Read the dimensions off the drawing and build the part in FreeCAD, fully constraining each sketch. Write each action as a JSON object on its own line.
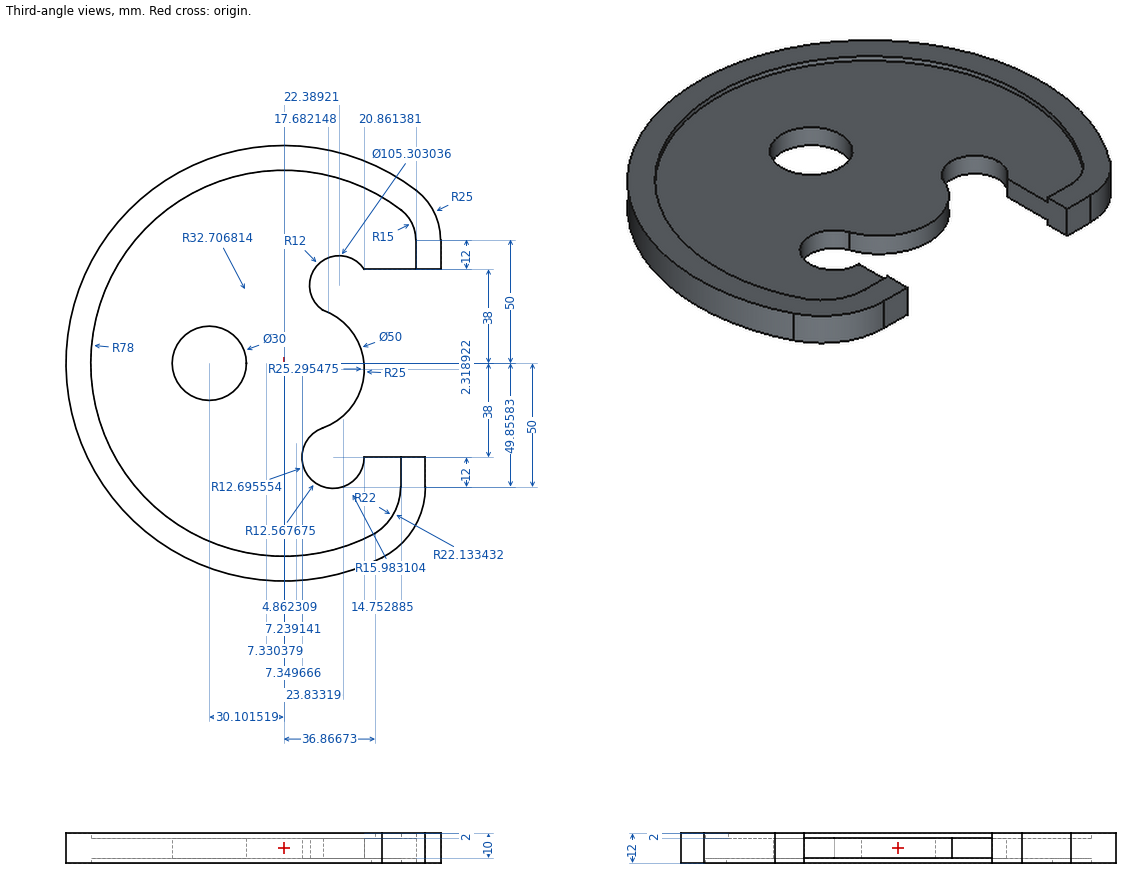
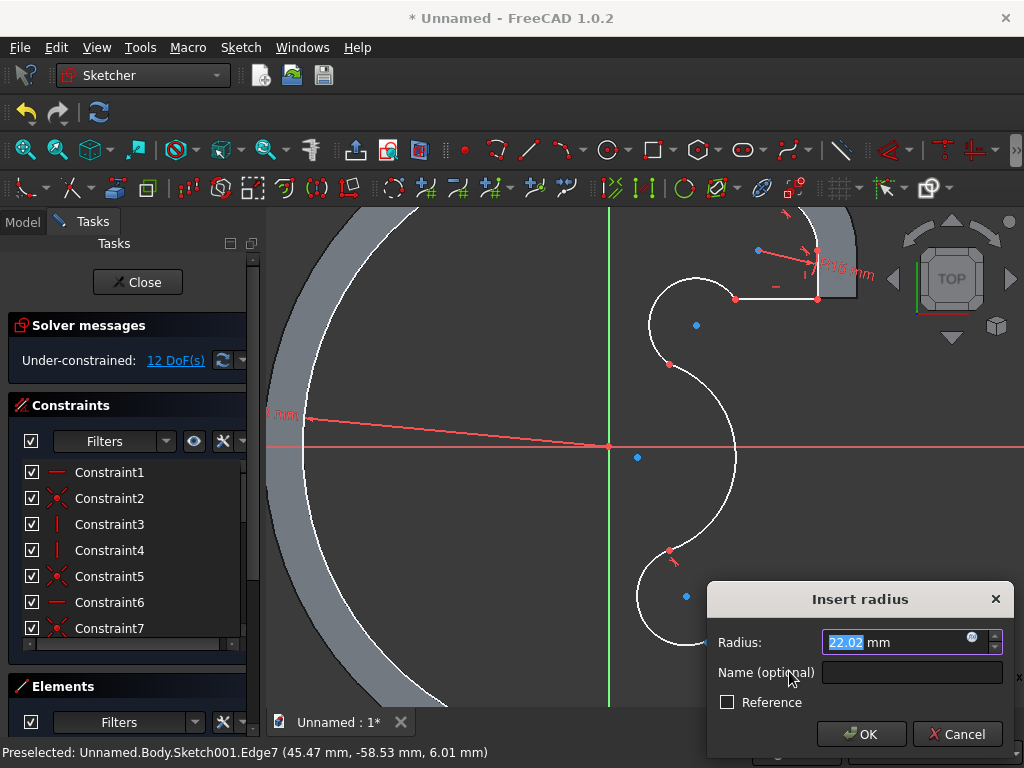
{"action": "type", "text": "22"}
{"action": "key", "text": "Return"}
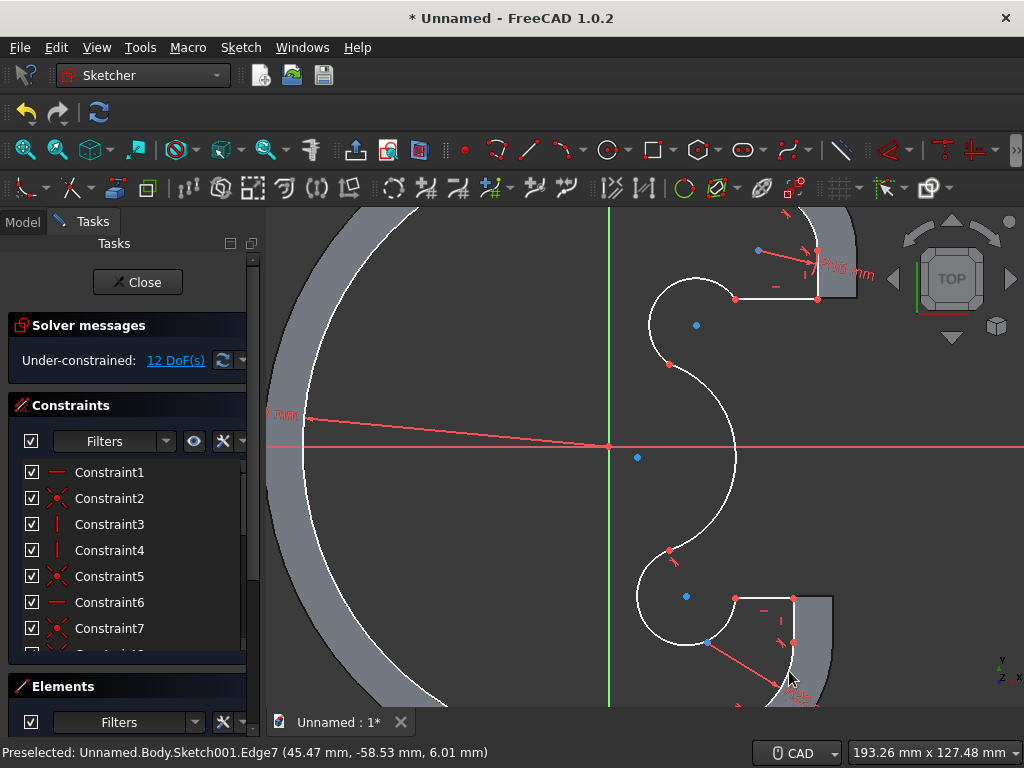
{"action": "left_click", "coordinate": [637, 600]}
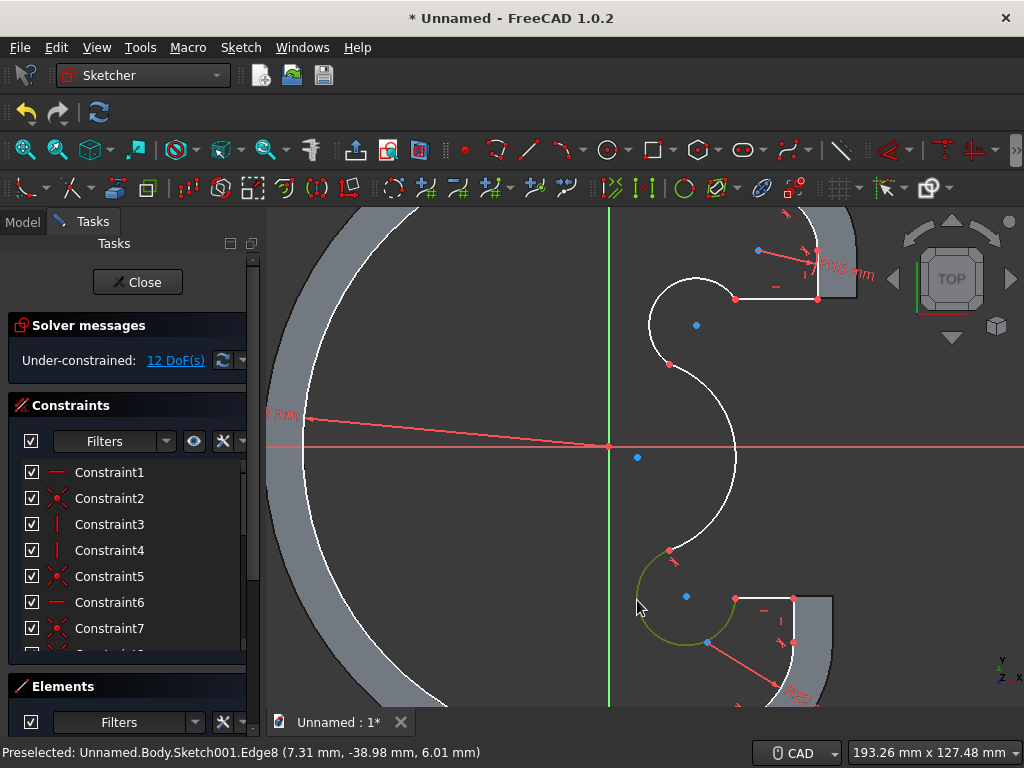
{"action": "key", "text": "k r"}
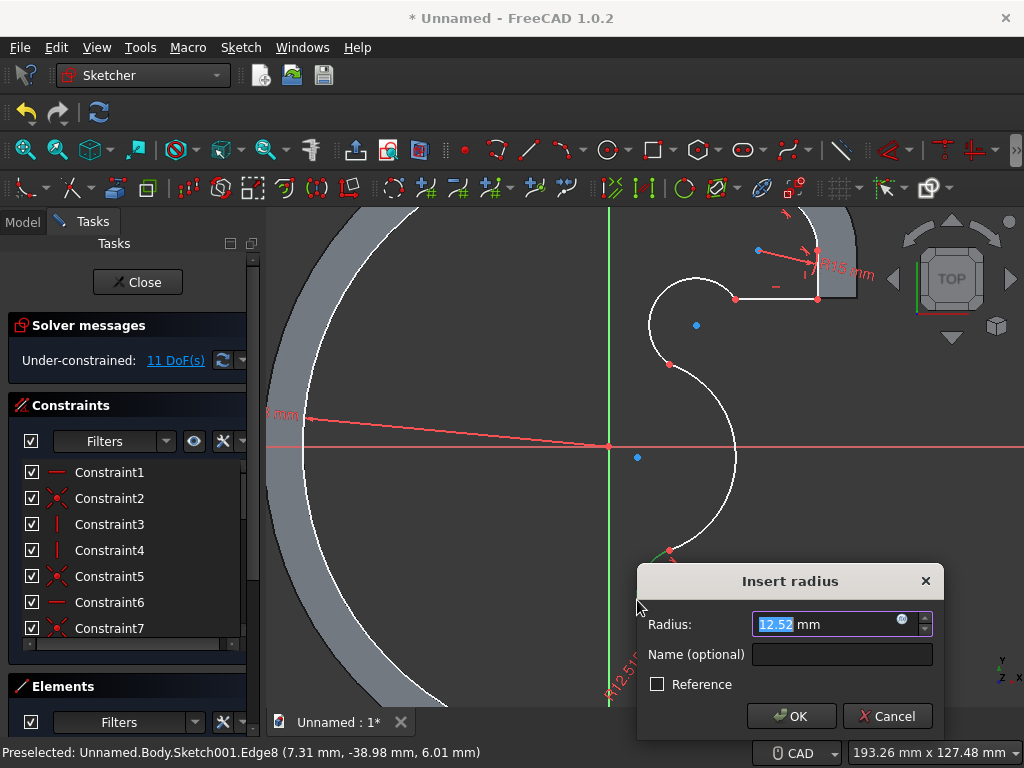
{"action": "type", "text": "12.567675"}
{"action": "key", "text": "Return"}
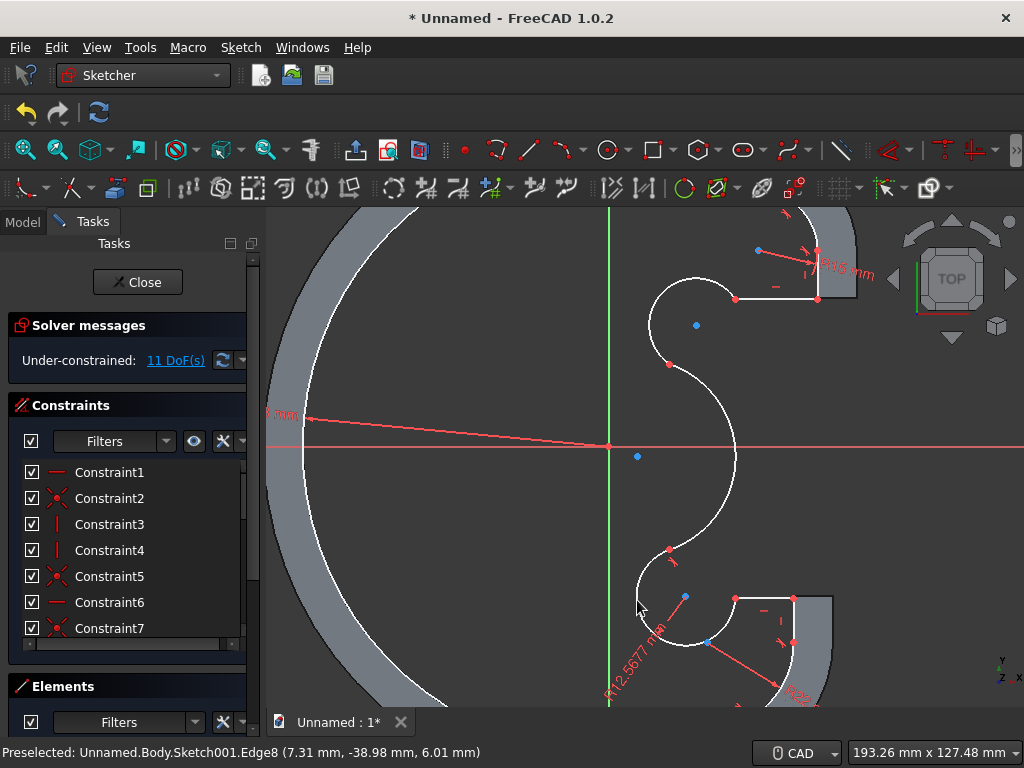
{"action": "left_click", "coordinate": [724, 504]}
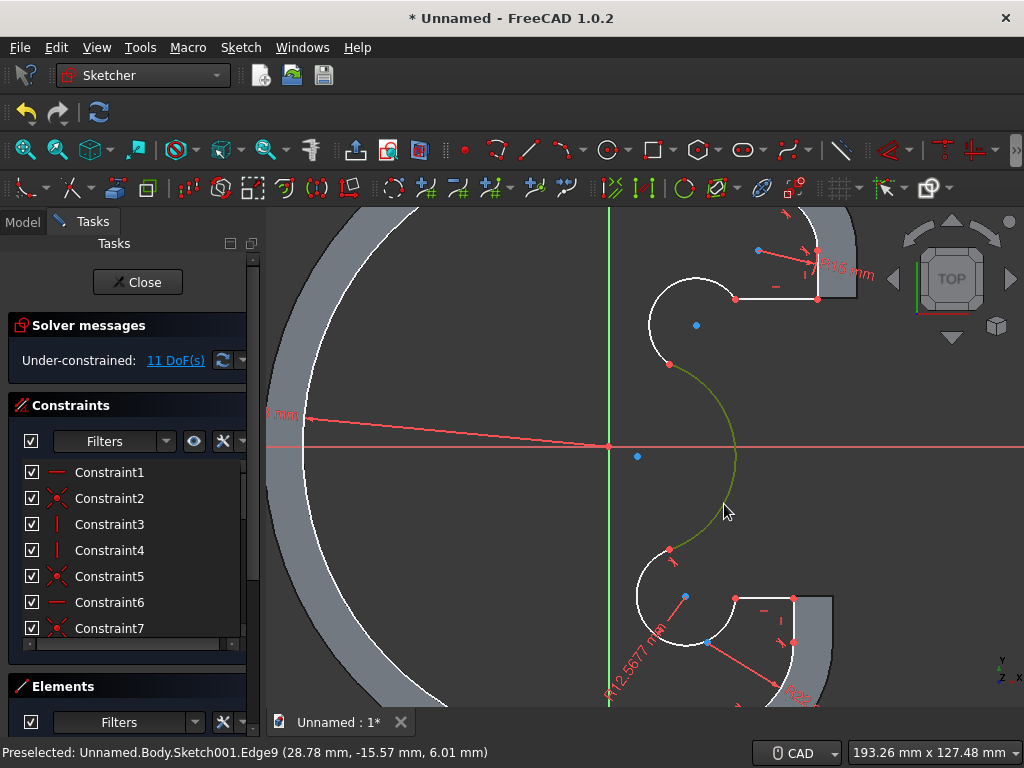
{"action": "key", "text": "k r"}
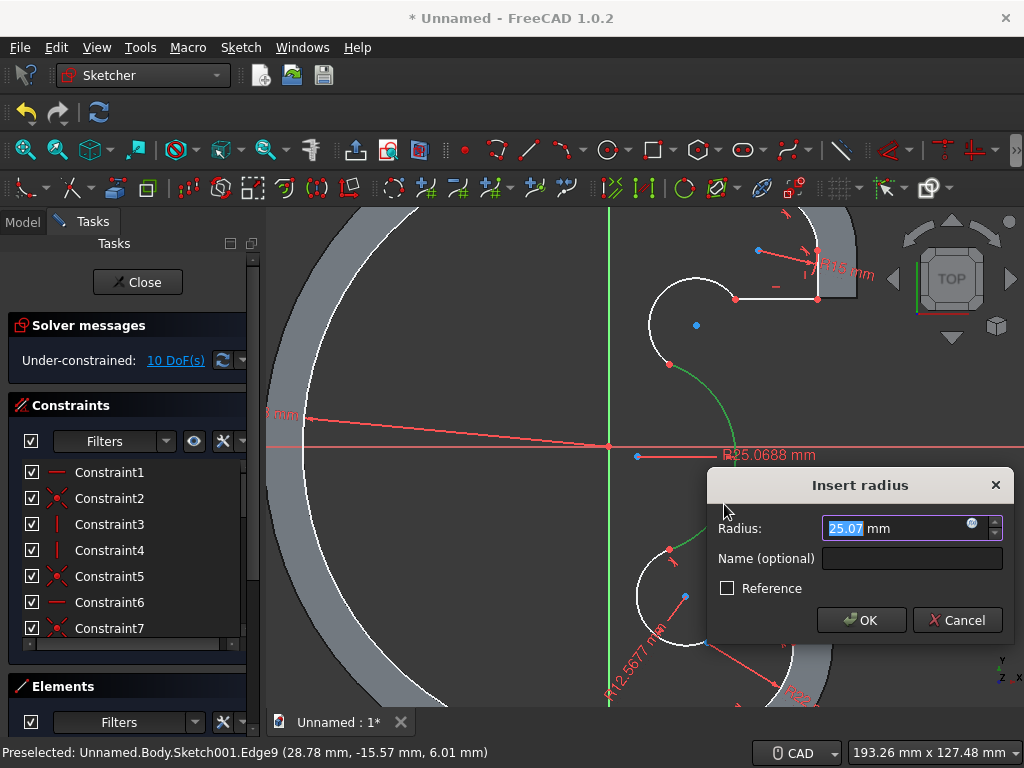
{"action": "type", "text": "25.295475"}
{"action": "key", "text": "Return"}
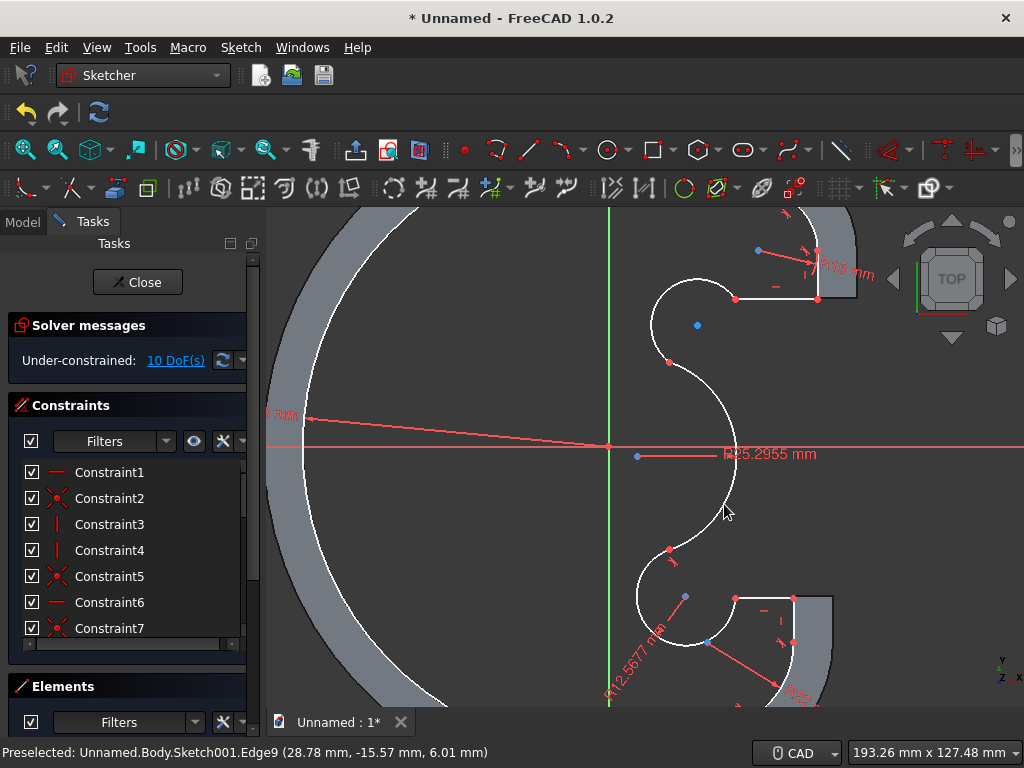
{"action": "left_click", "coordinate": [694, 279]}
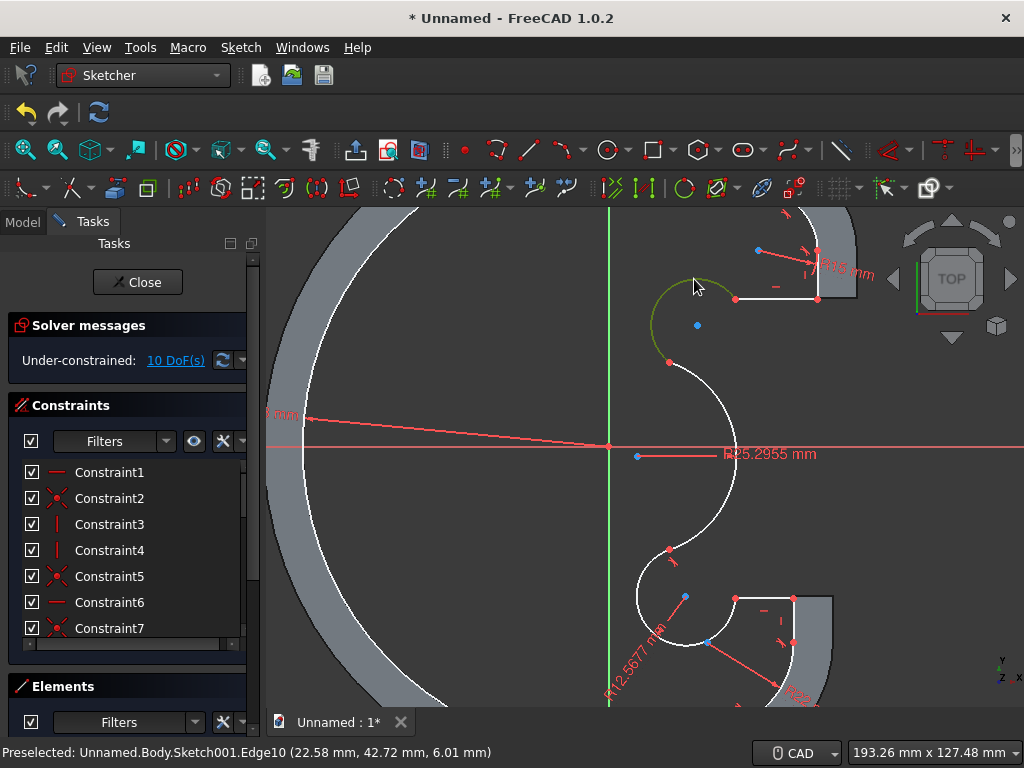
{"action": "left_click", "coordinate": [912, 150]}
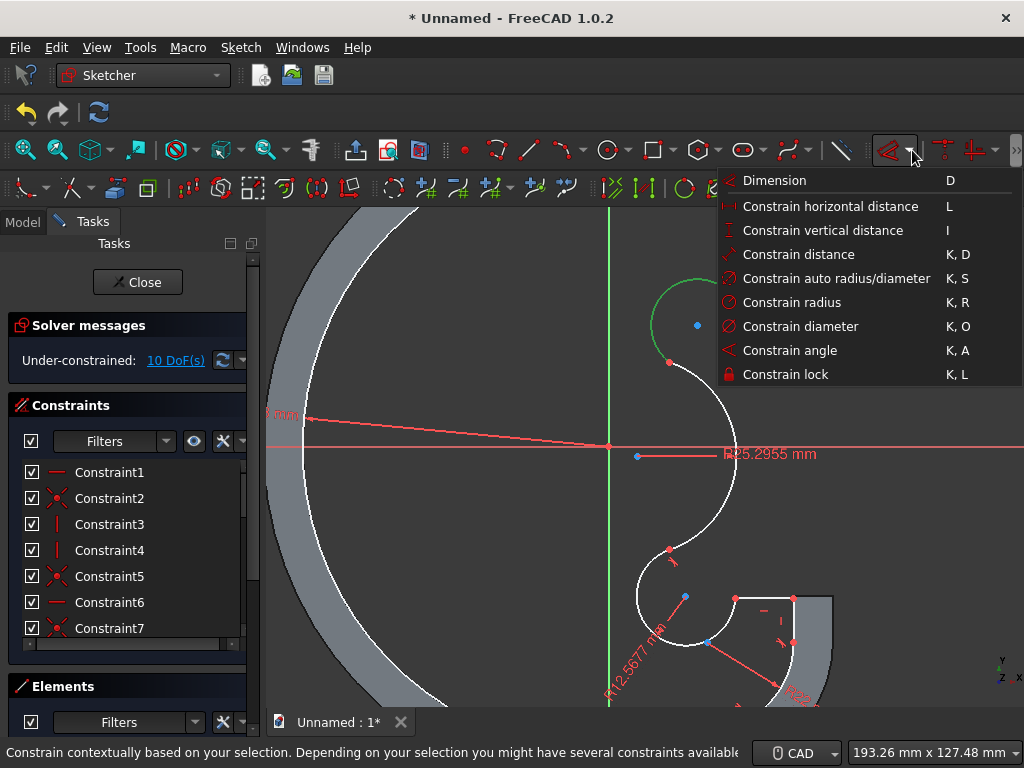
{"action": "left_click", "coordinate": [870, 302]}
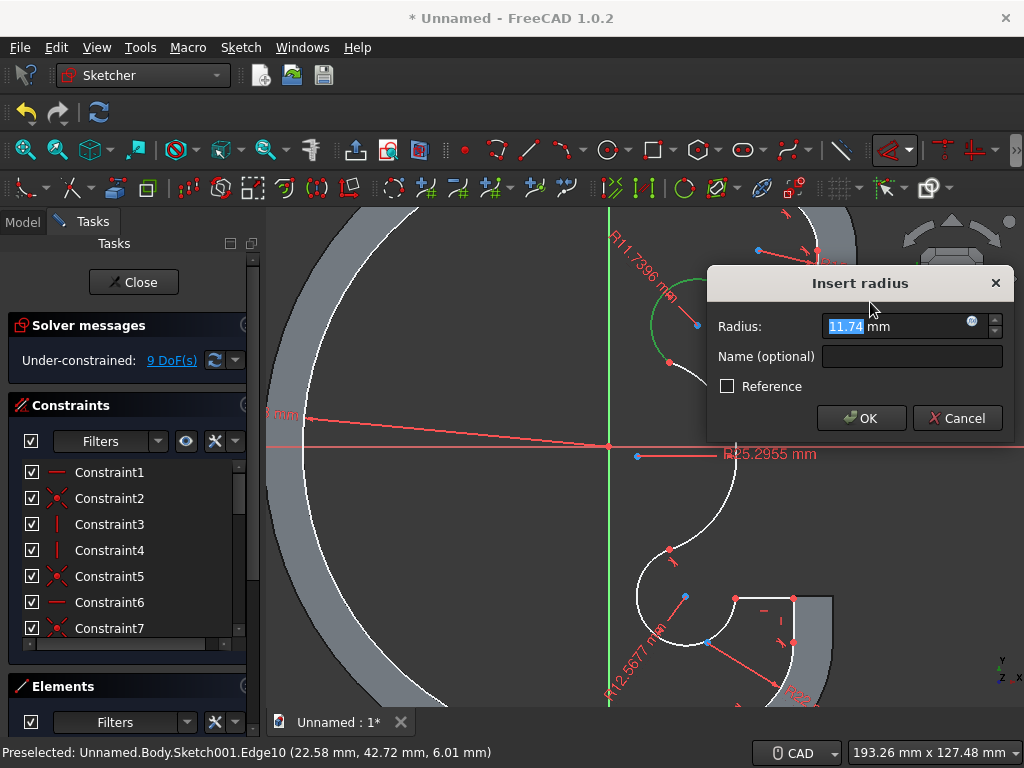
{"action": "type", "text": "12"}
{"action": "key", "text": "Return"}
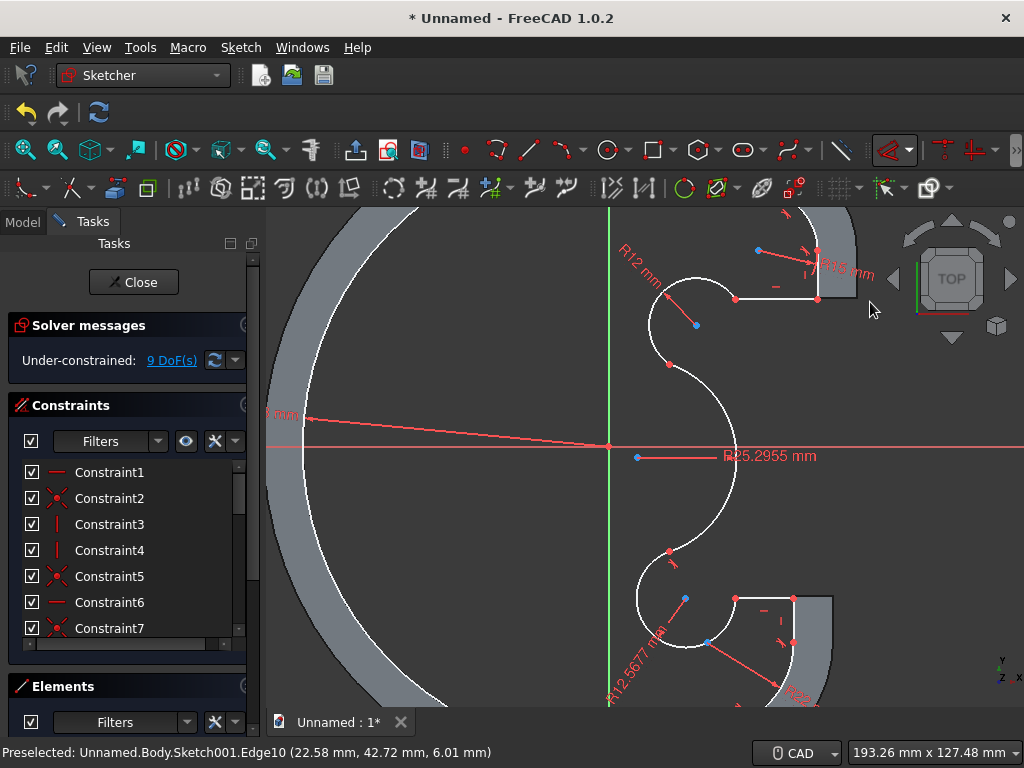
{"action": "left_click", "coordinate": [818, 285]}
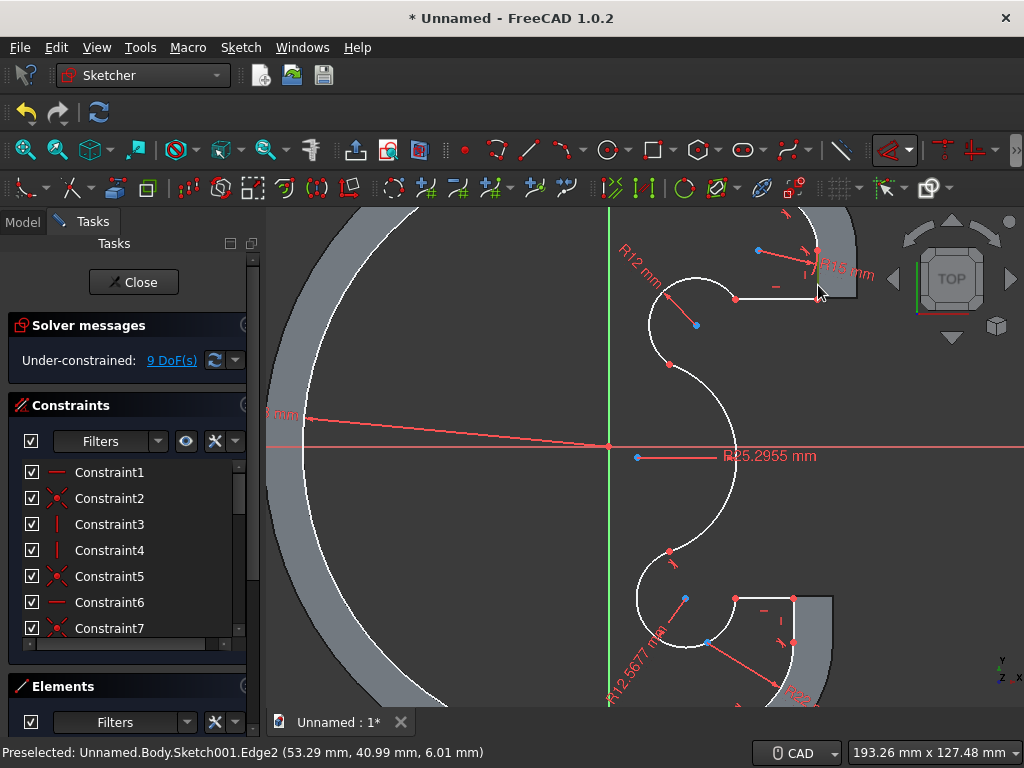
{"action": "key", "text": "i"}